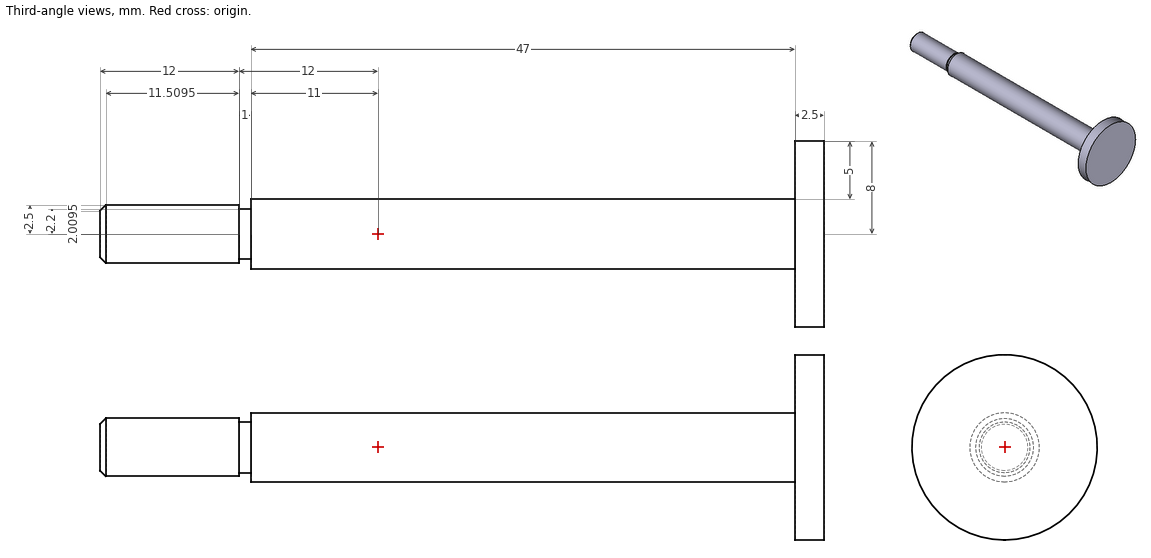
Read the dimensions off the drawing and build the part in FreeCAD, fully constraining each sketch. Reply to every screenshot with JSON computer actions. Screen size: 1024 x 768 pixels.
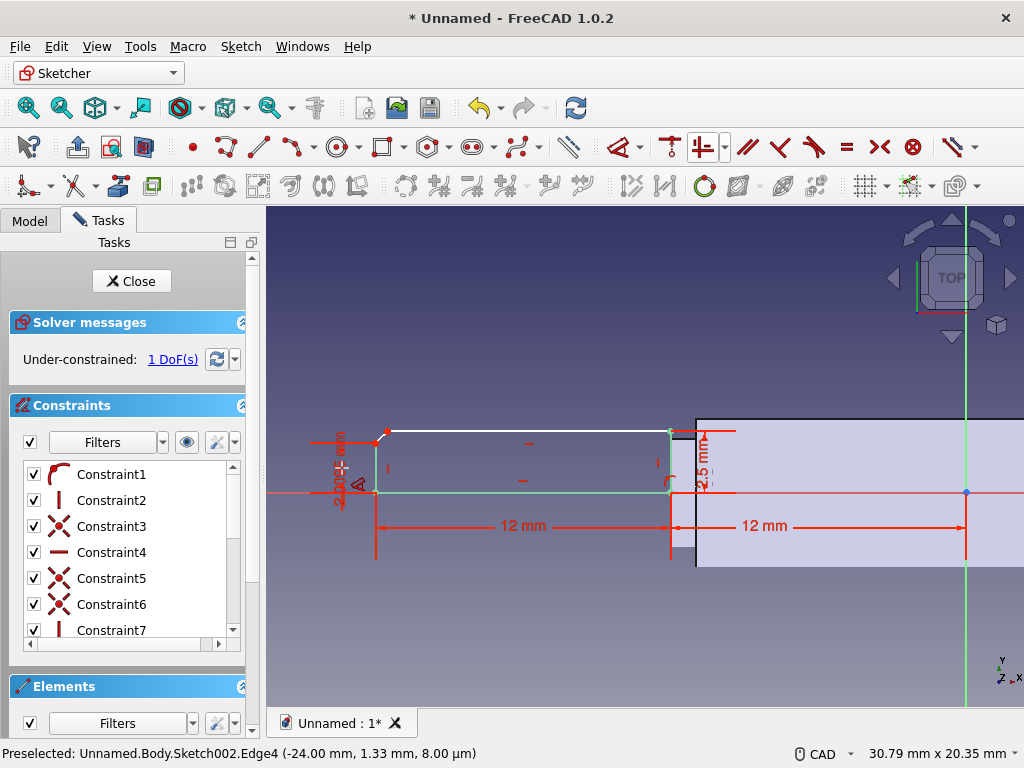
{"action": "left_click", "coordinate": [586, 431]}
{"action": "left_click", "coordinate": [529, 397]}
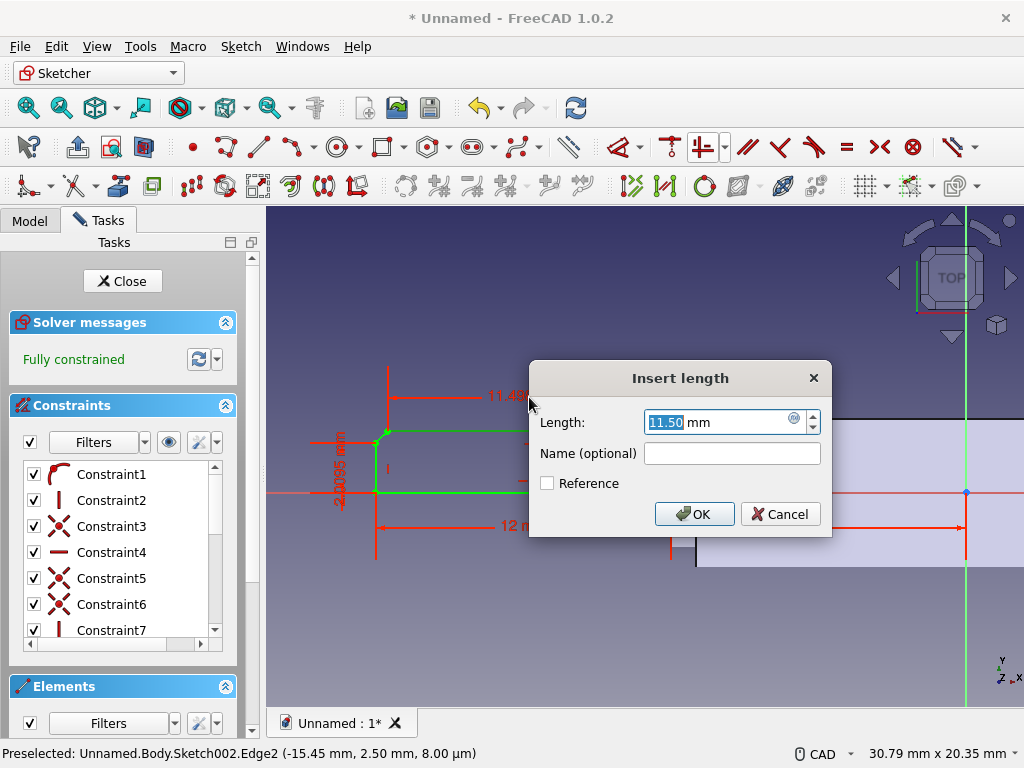
{"action": "type", "text": "11.5095"}
{"action": "key", "text": "Return"}
{"action": "key", "text": "Escape"}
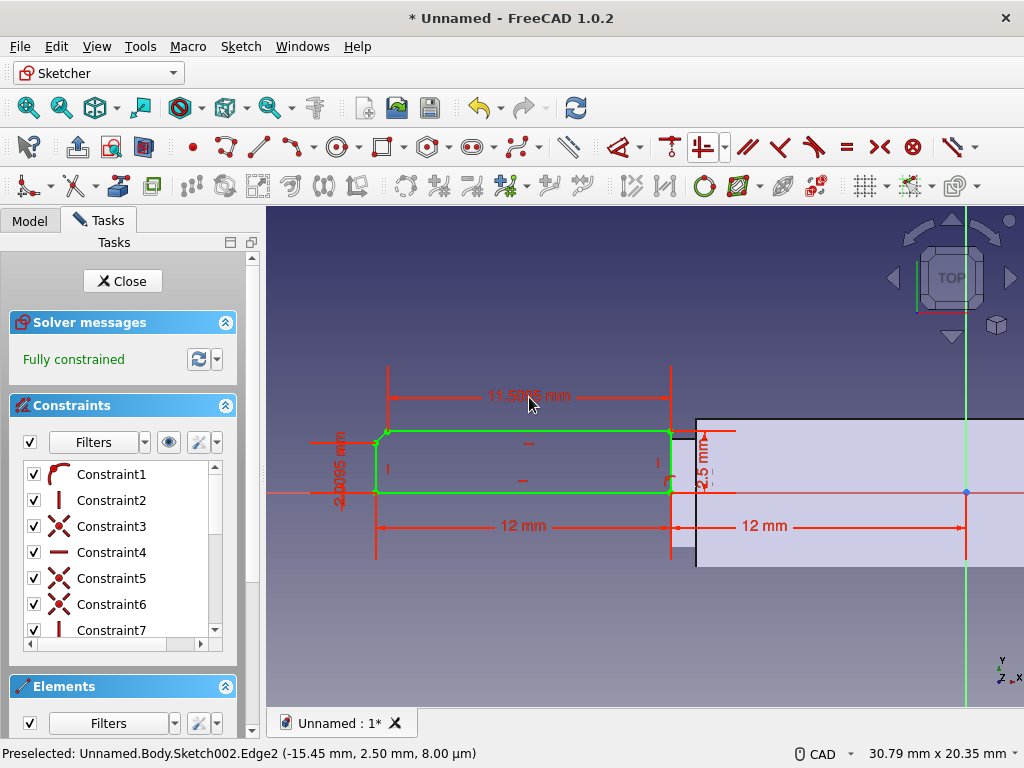
{"action": "left_click", "coordinate": [123, 281]}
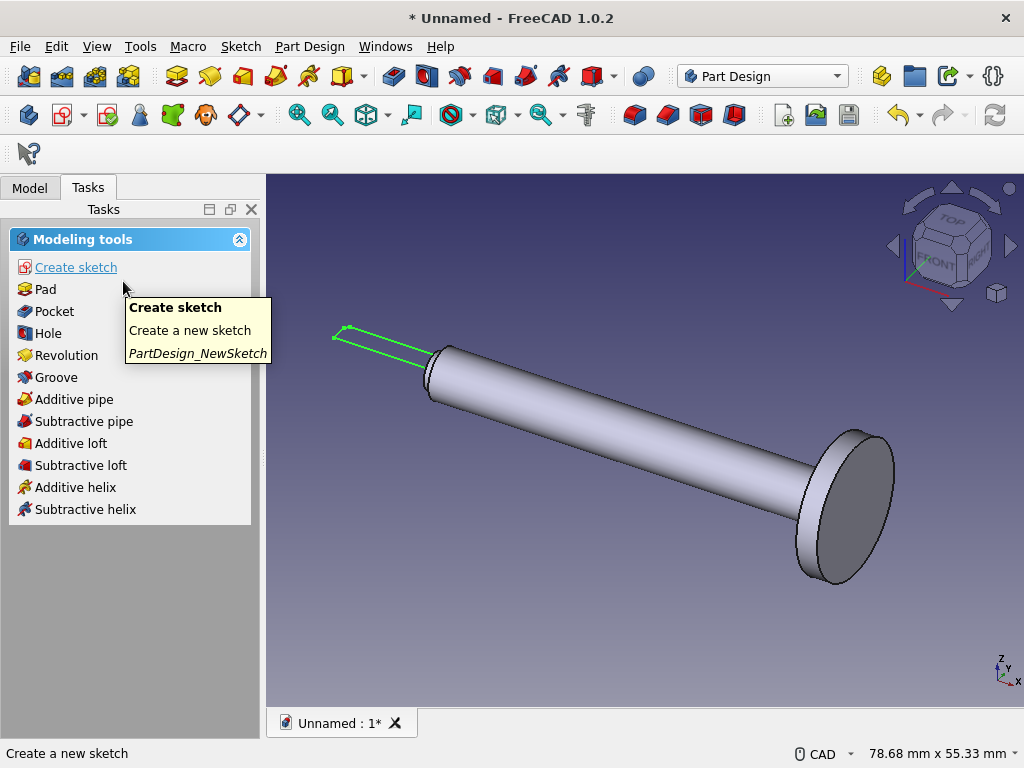
{"action": "left_click", "coordinate": [210, 76]}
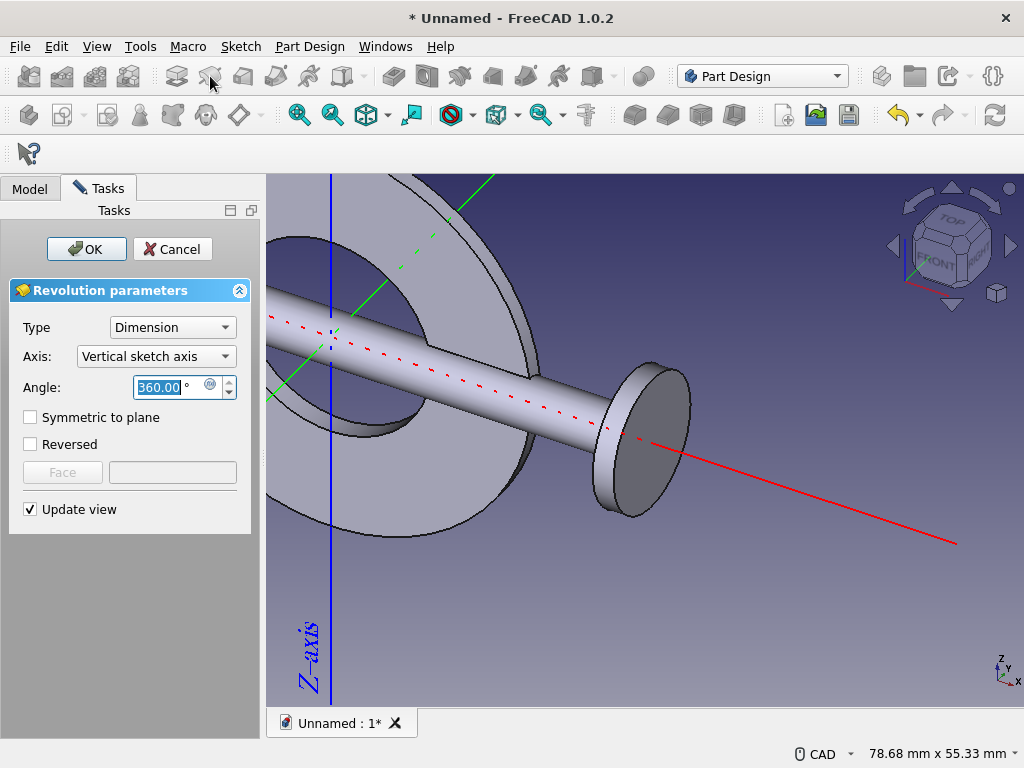
{"action": "left_click", "coordinate": [157, 356]}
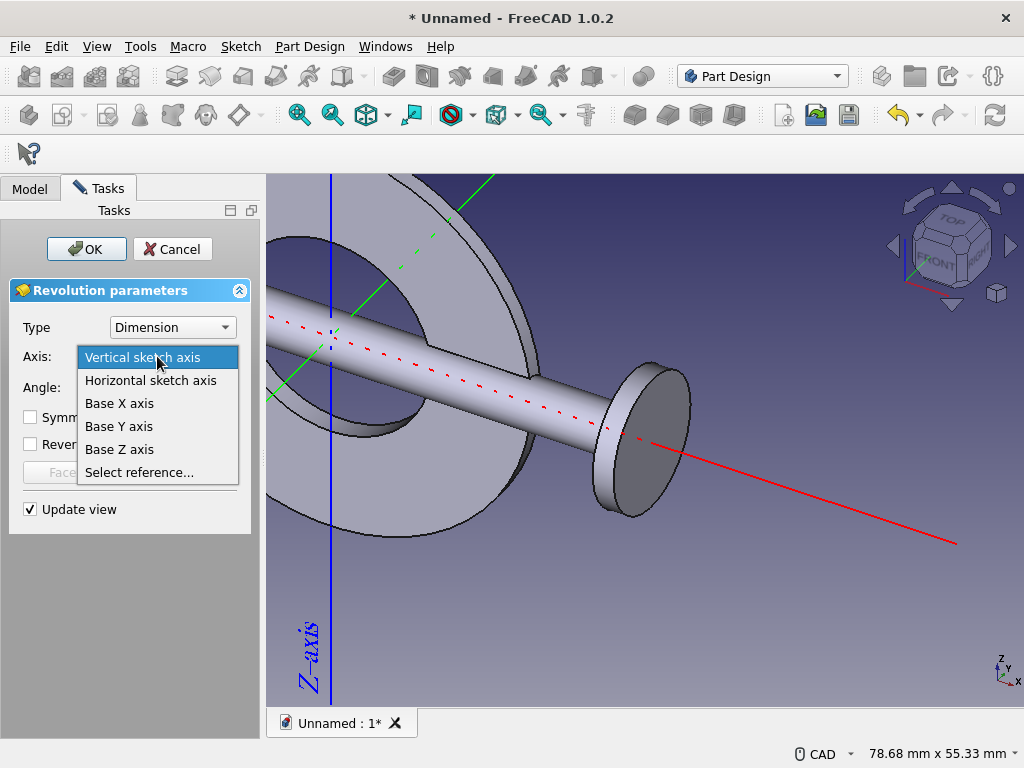
{"action": "left_click", "coordinate": [156, 380]}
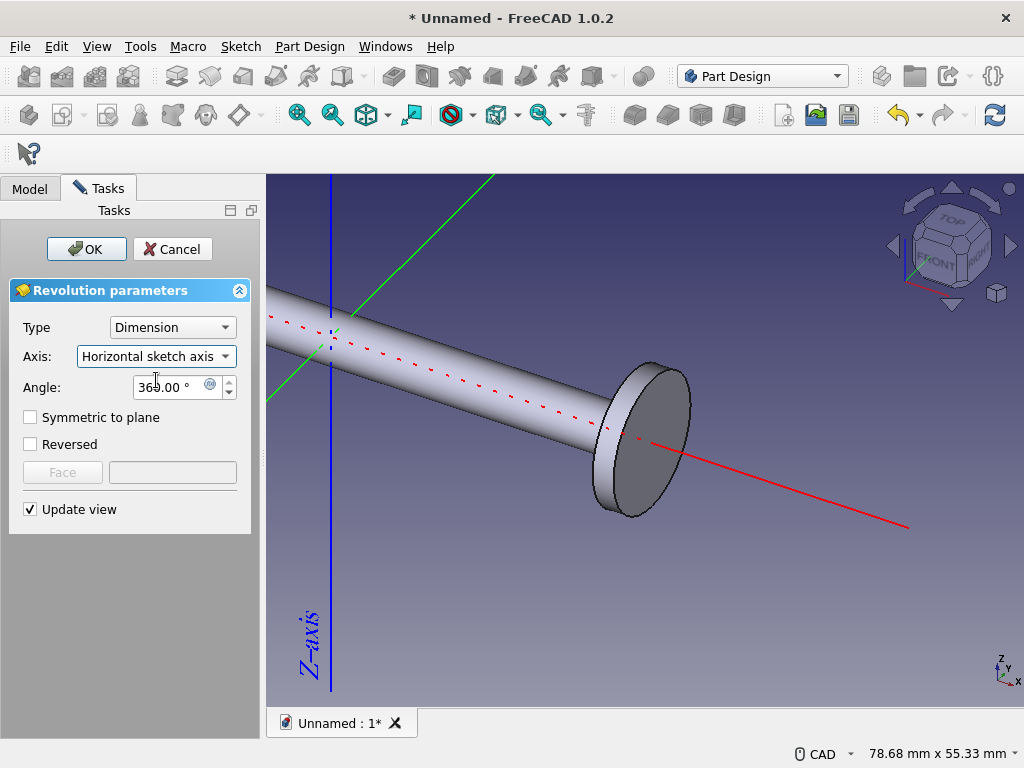
{"action": "left_click", "coordinate": [87, 249]}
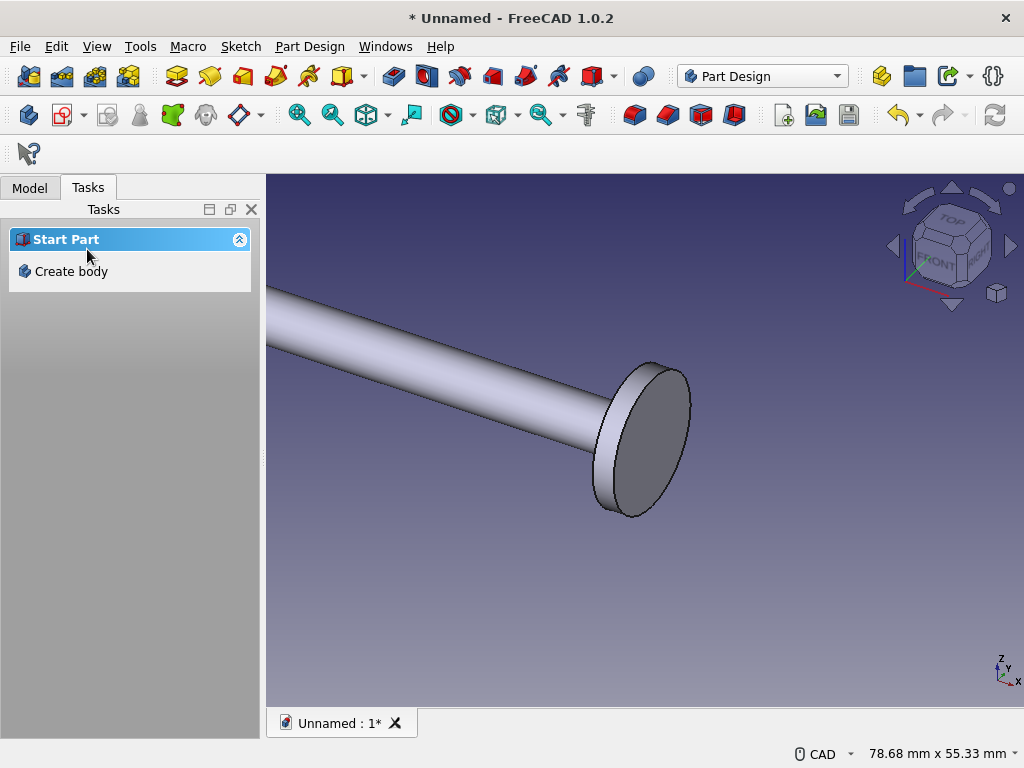
{"action": "key", "text": "0"}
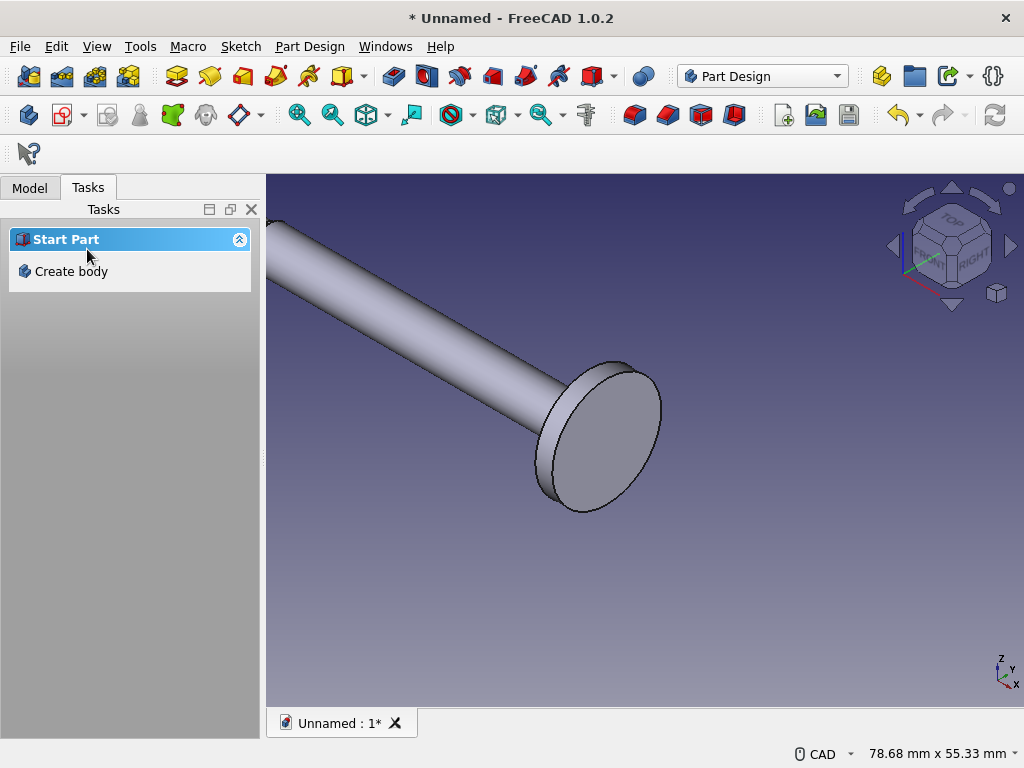
{"action": "left_click", "coordinate": [300, 116]}